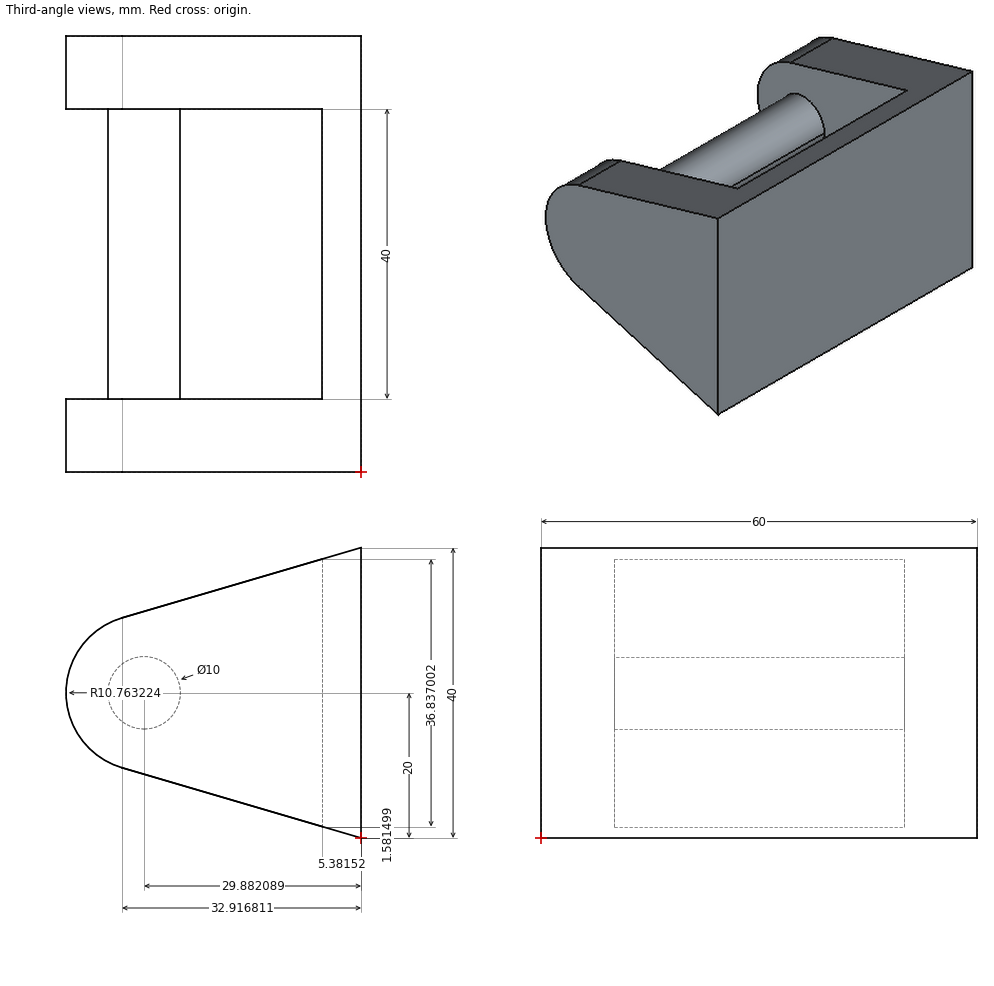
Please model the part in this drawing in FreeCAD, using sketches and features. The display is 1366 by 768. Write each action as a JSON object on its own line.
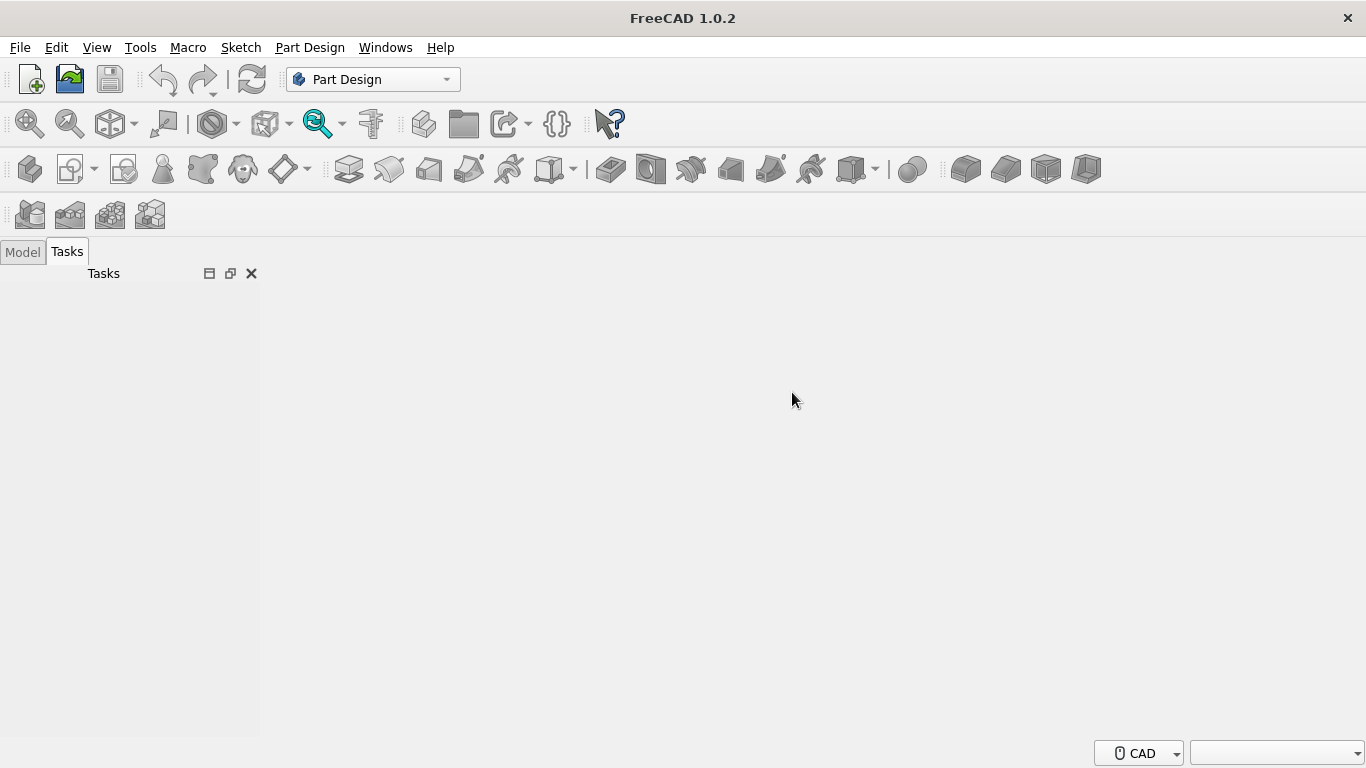
{"action": "left_click", "coordinate": [30, 80]}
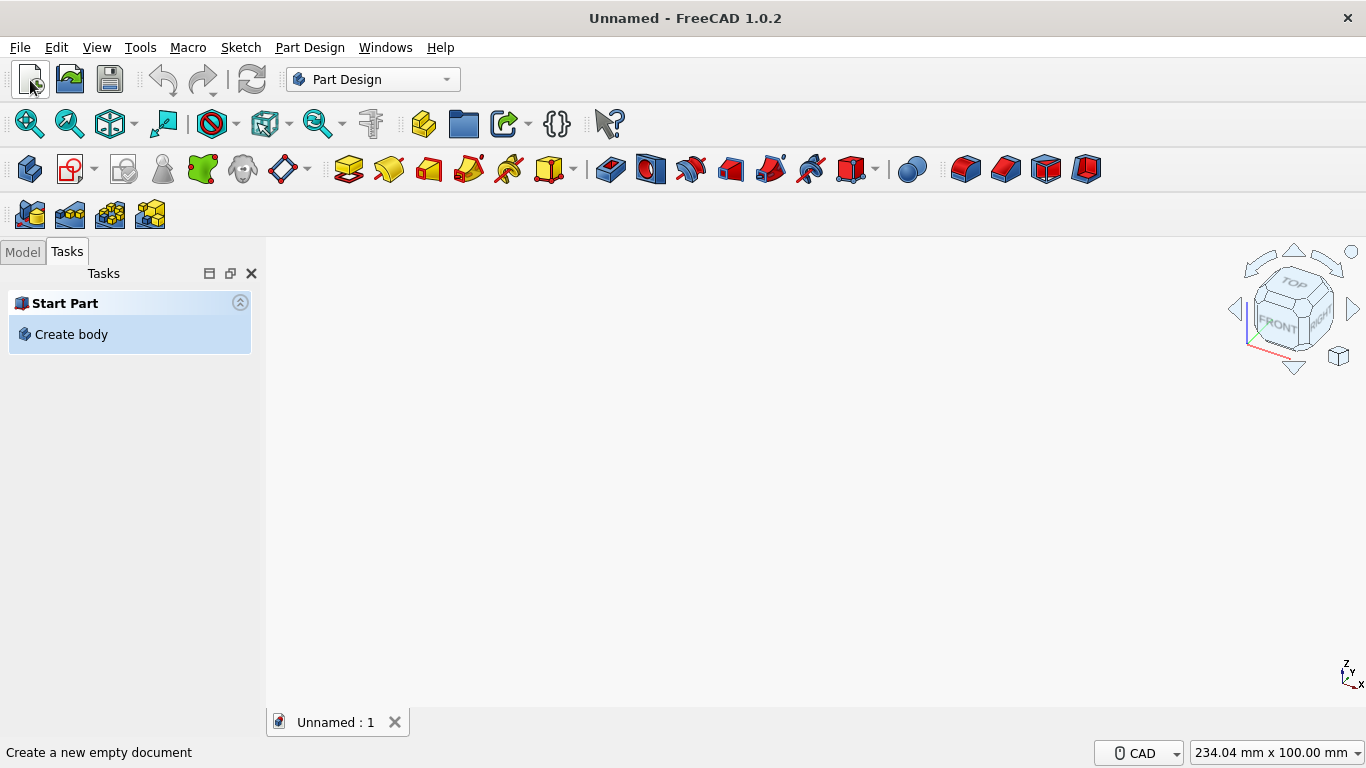
{"action": "left_click", "coordinate": [70, 170]}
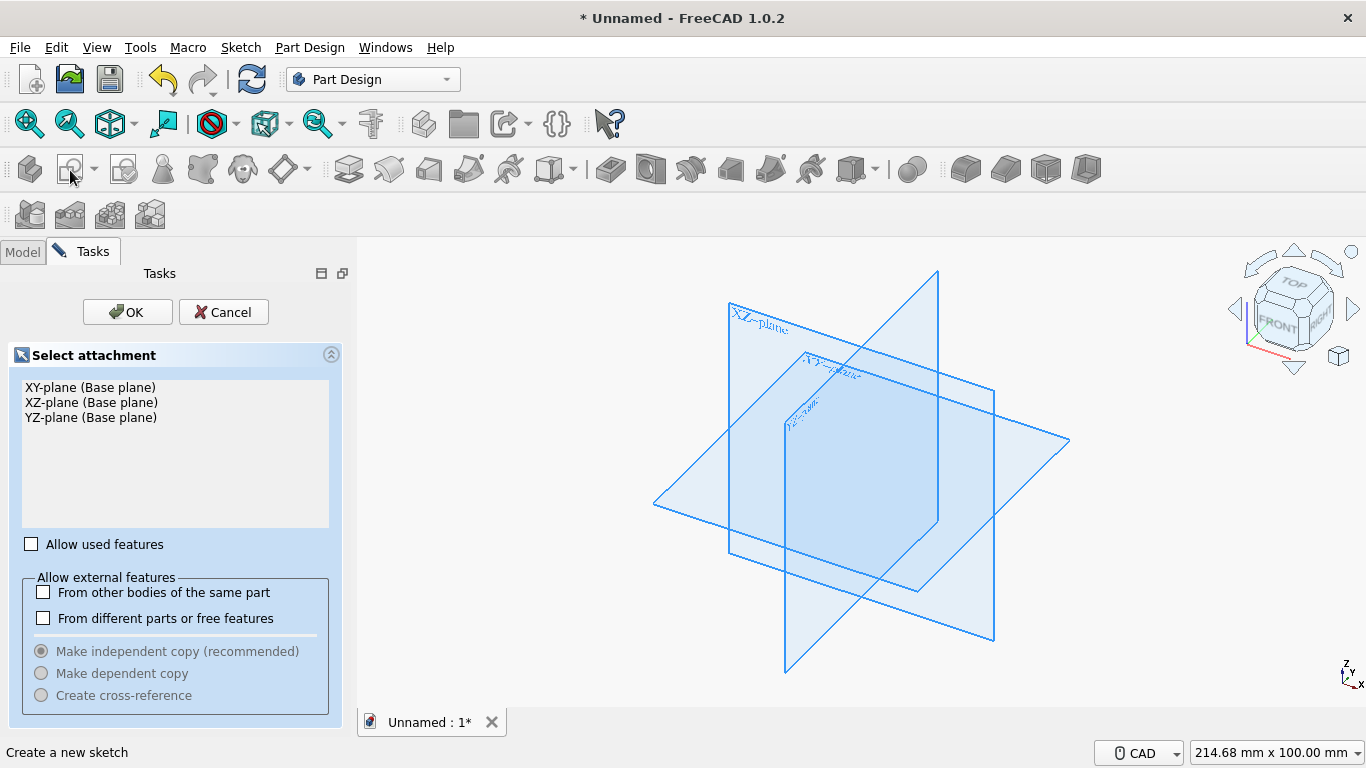
{"action": "left_click", "coordinate": [82, 402]}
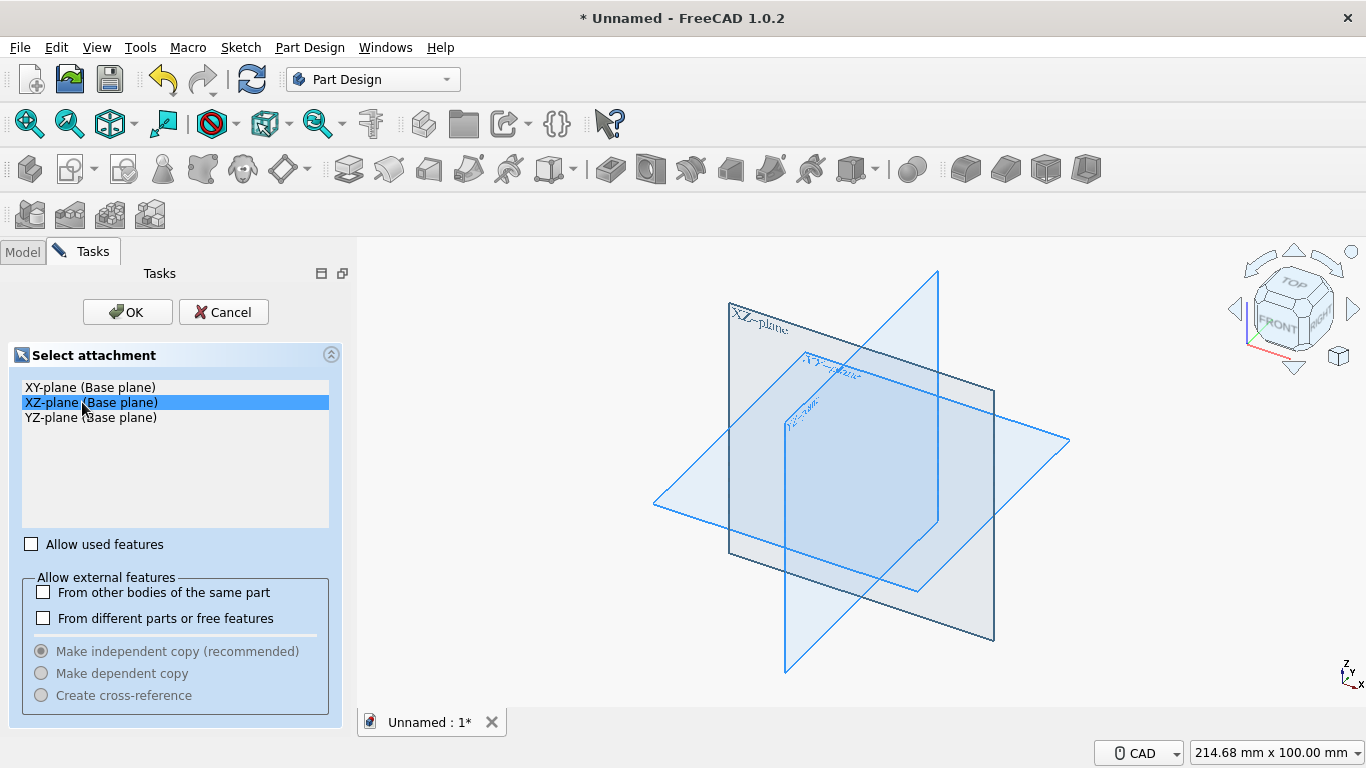
{"action": "left_click", "coordinate": [128, 312]}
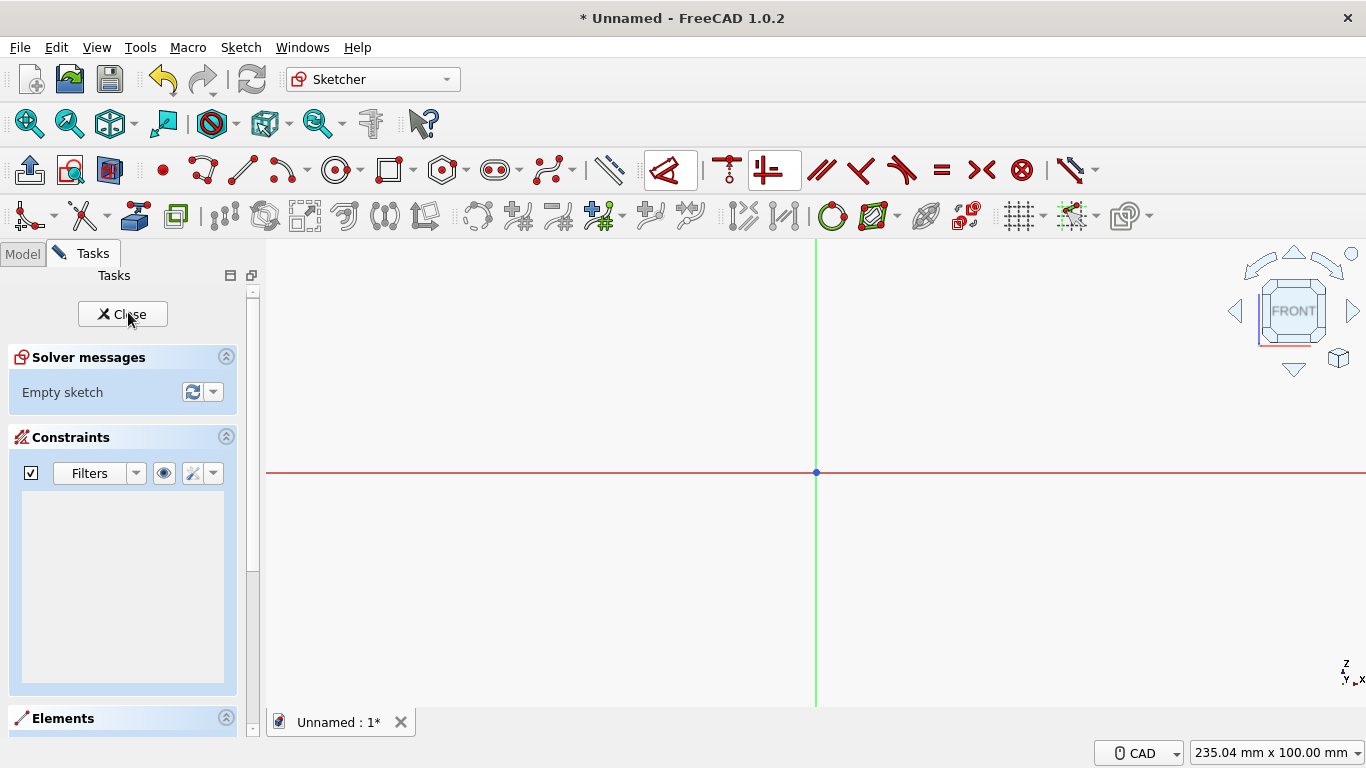
{"action": "scroll", "coordinate": [667, 267], "scroll_direction": "up", "scroll_amount": 2}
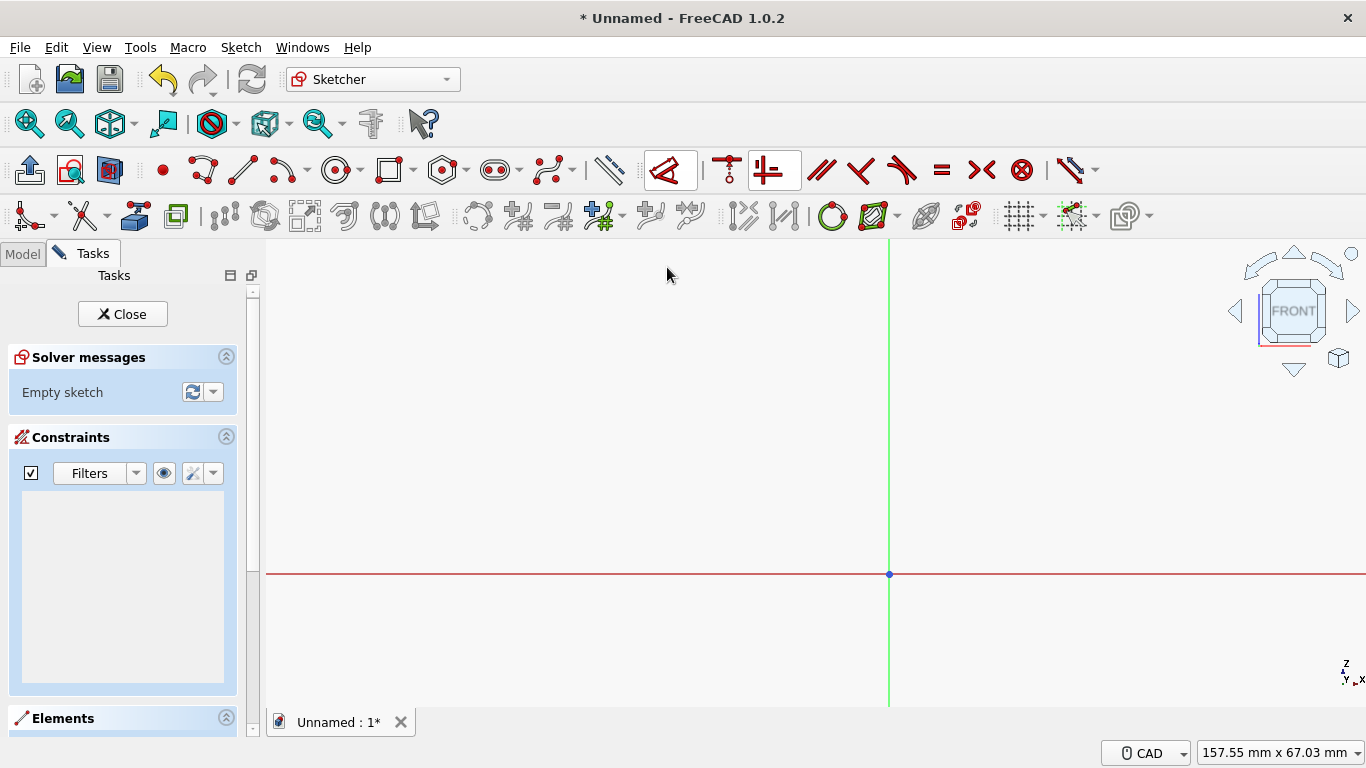
{"action": "left_click", "coordinate": [204, 170]}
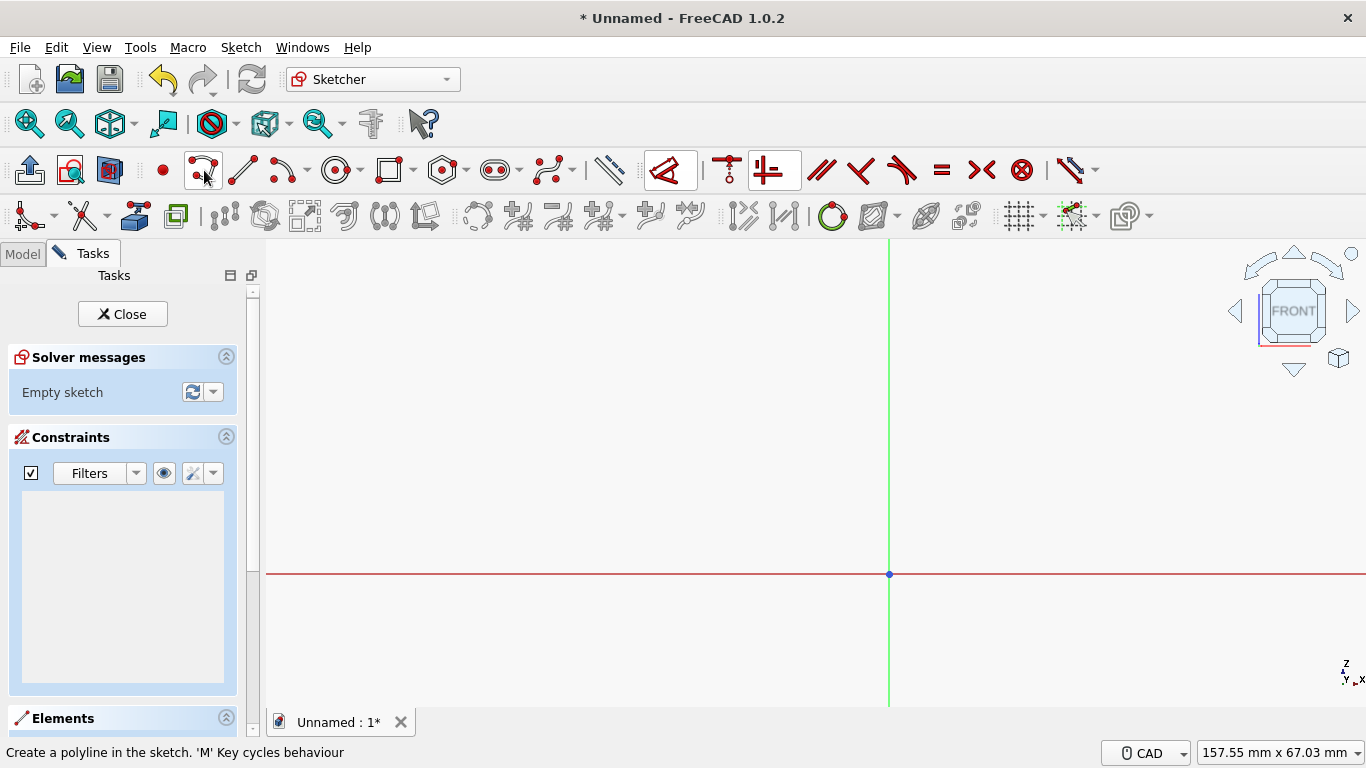
{"action": "left_click", "coordinate": [659, 363]}
{"action": "left_click", "coordinate": [889, 295]}
{"action": "left_click", "coordinate": [889, 574]}
{"action": "left_click", "coordinate": [659, 507]}
{"action": "right_click", "coordinate": [659, 507]}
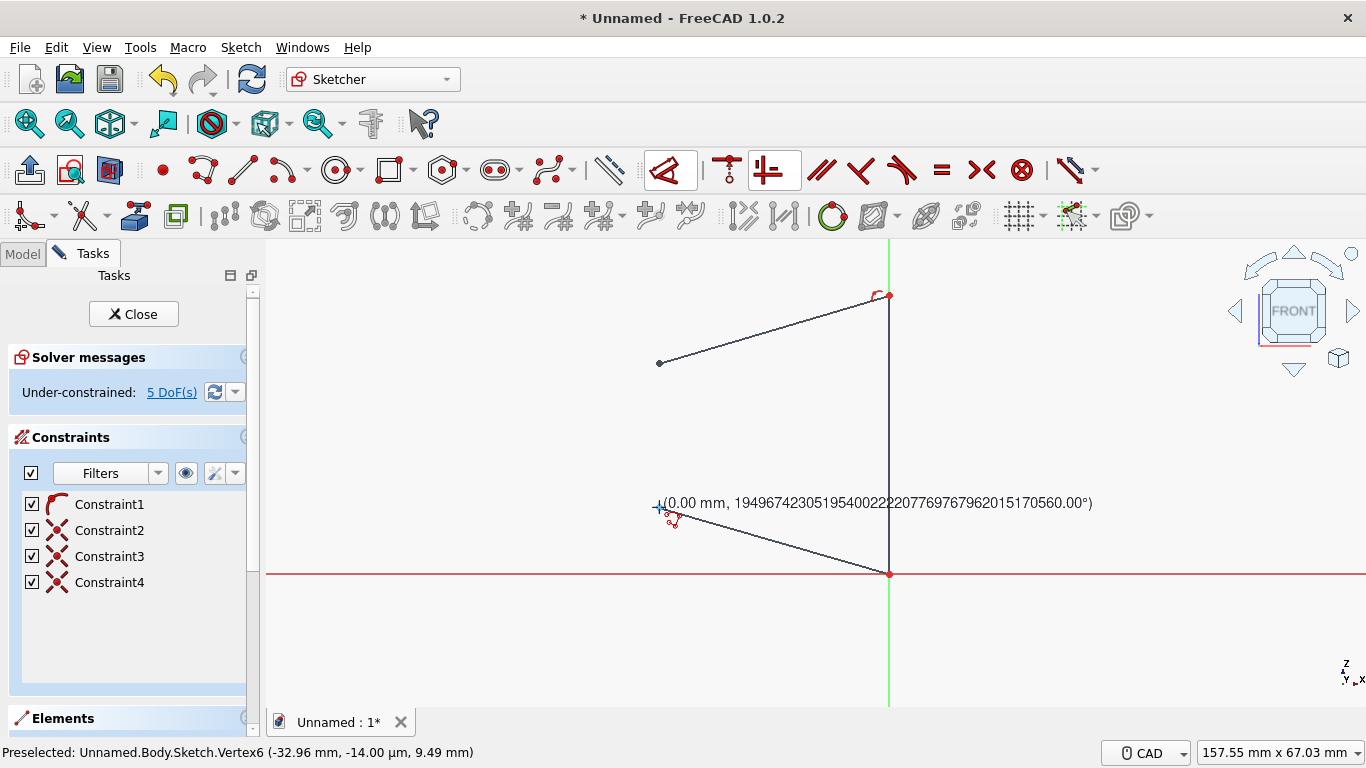
{"action": "key", "text": "g 3 a"}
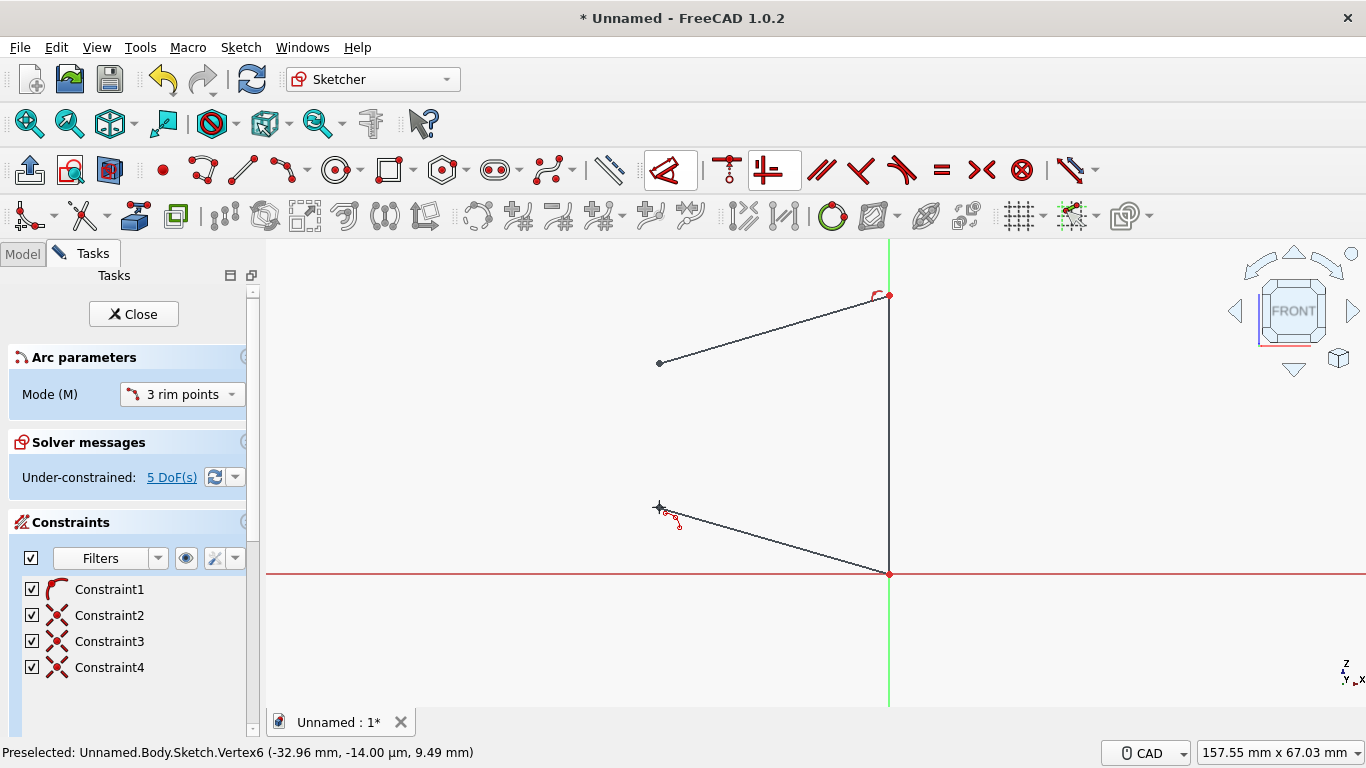
{"action": "left_click", "coordinate": [659, 508]}
{"action": "left_click", "coordinate": [659, 364]}
{"action": "left_click", "coordinate": [605, 435]}
{"action": "key", "text": "Escape"}